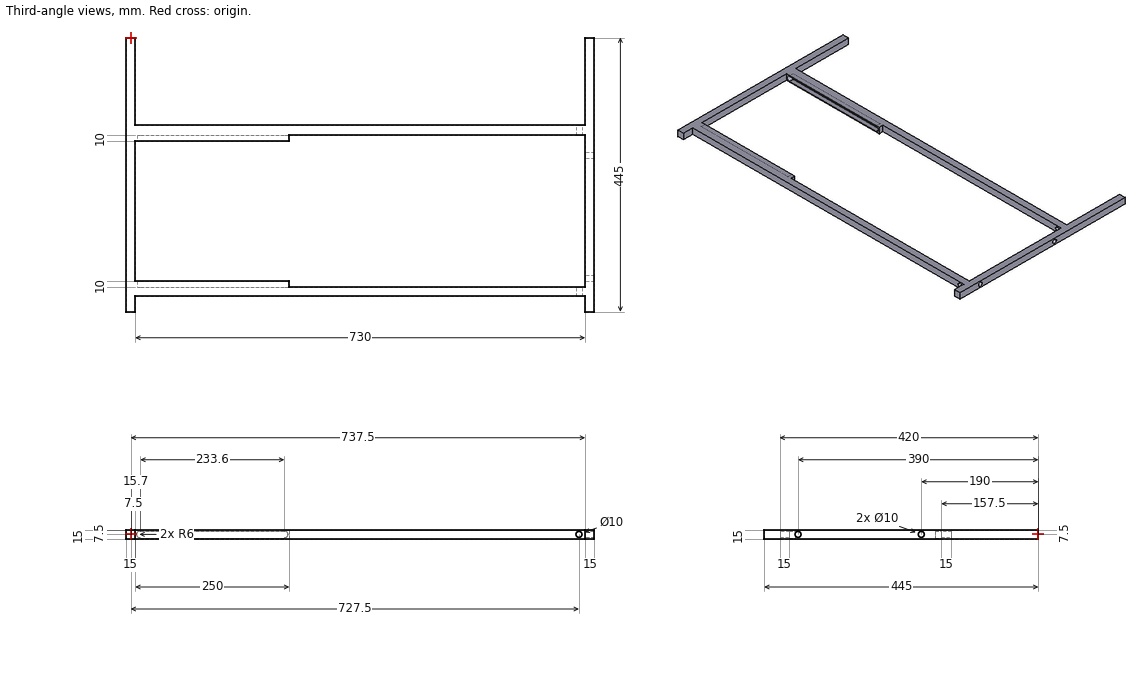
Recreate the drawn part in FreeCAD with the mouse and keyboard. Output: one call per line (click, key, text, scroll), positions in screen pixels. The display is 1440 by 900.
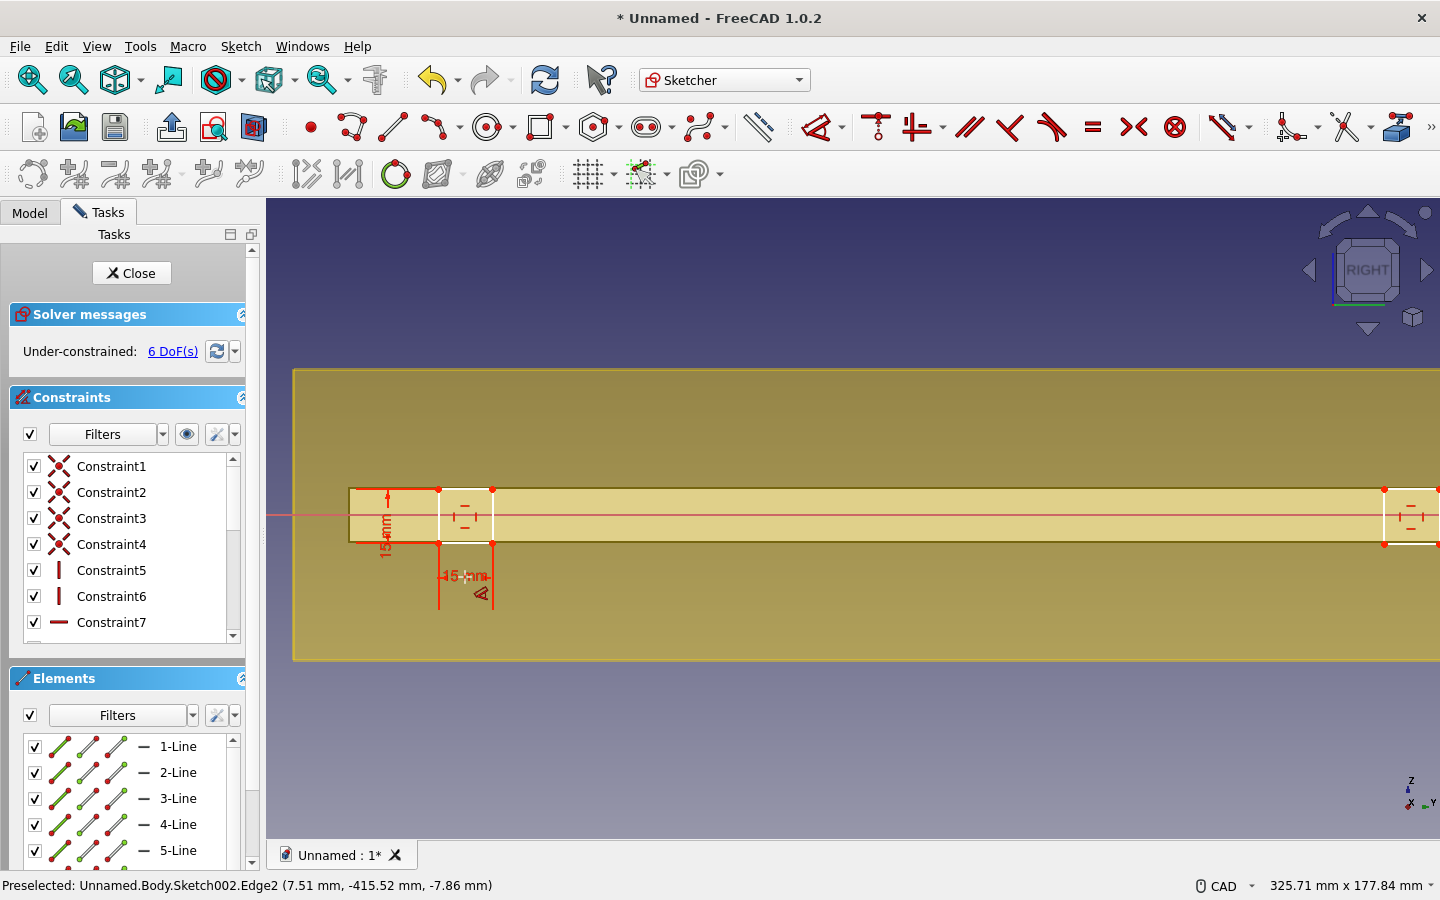
scroll(449, 521, down, 4)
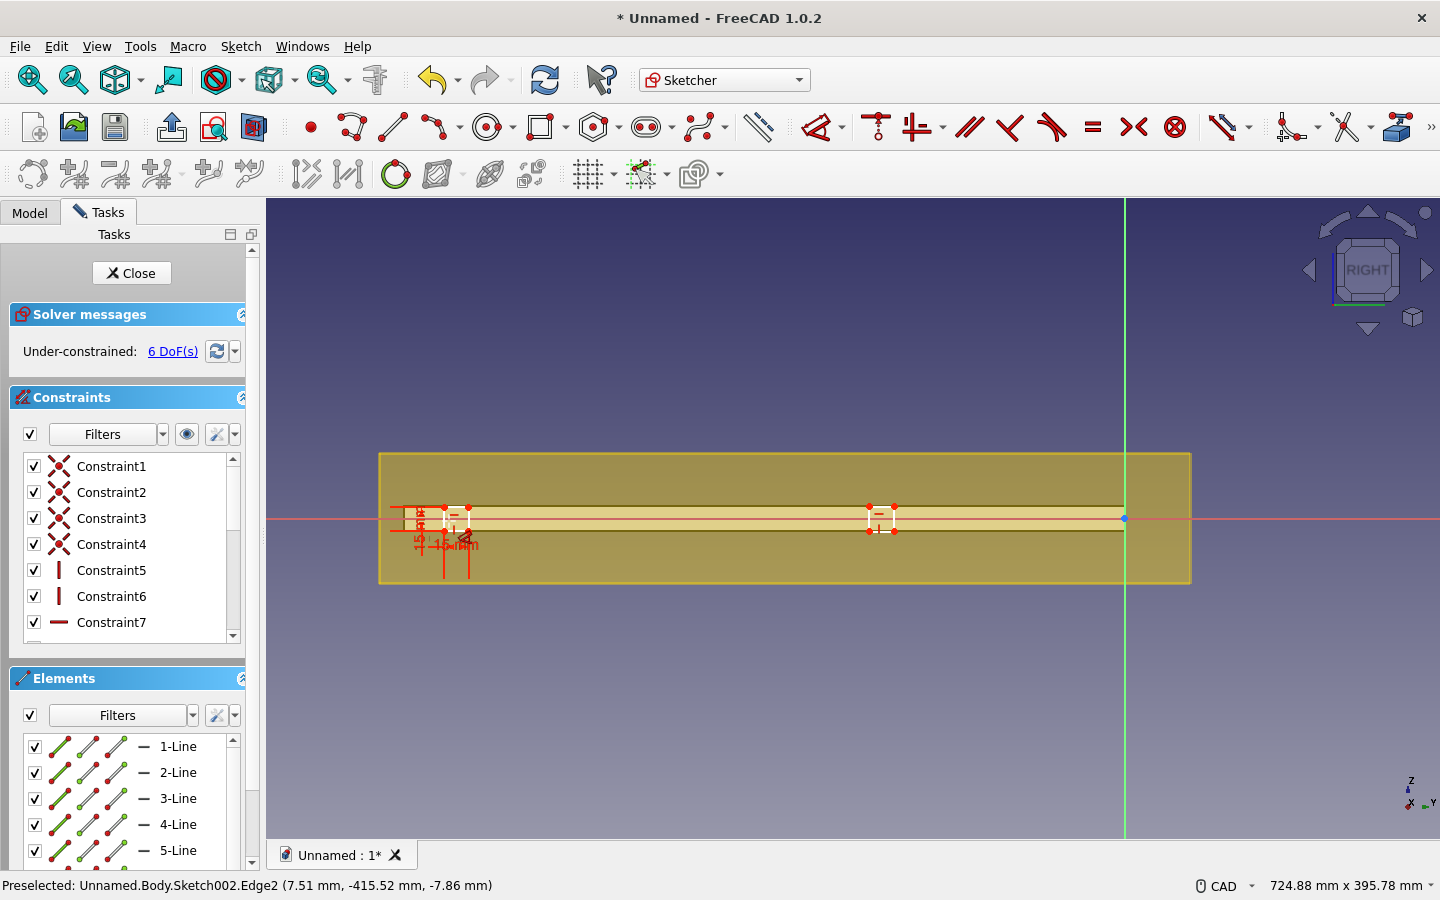
scroll(869, 514, up, 6)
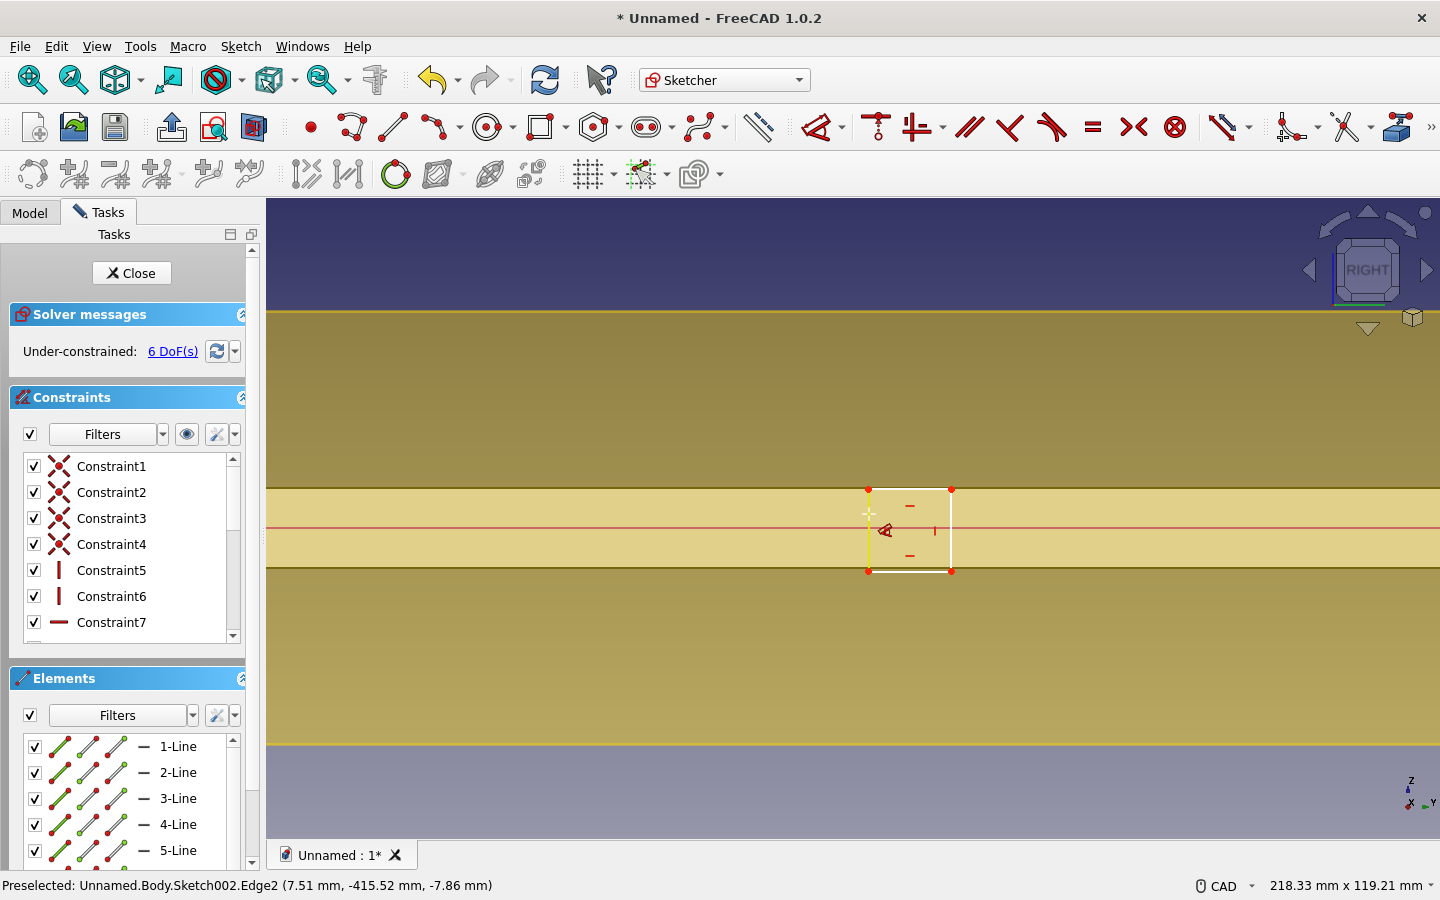
click(869, 514)
click(903, 512)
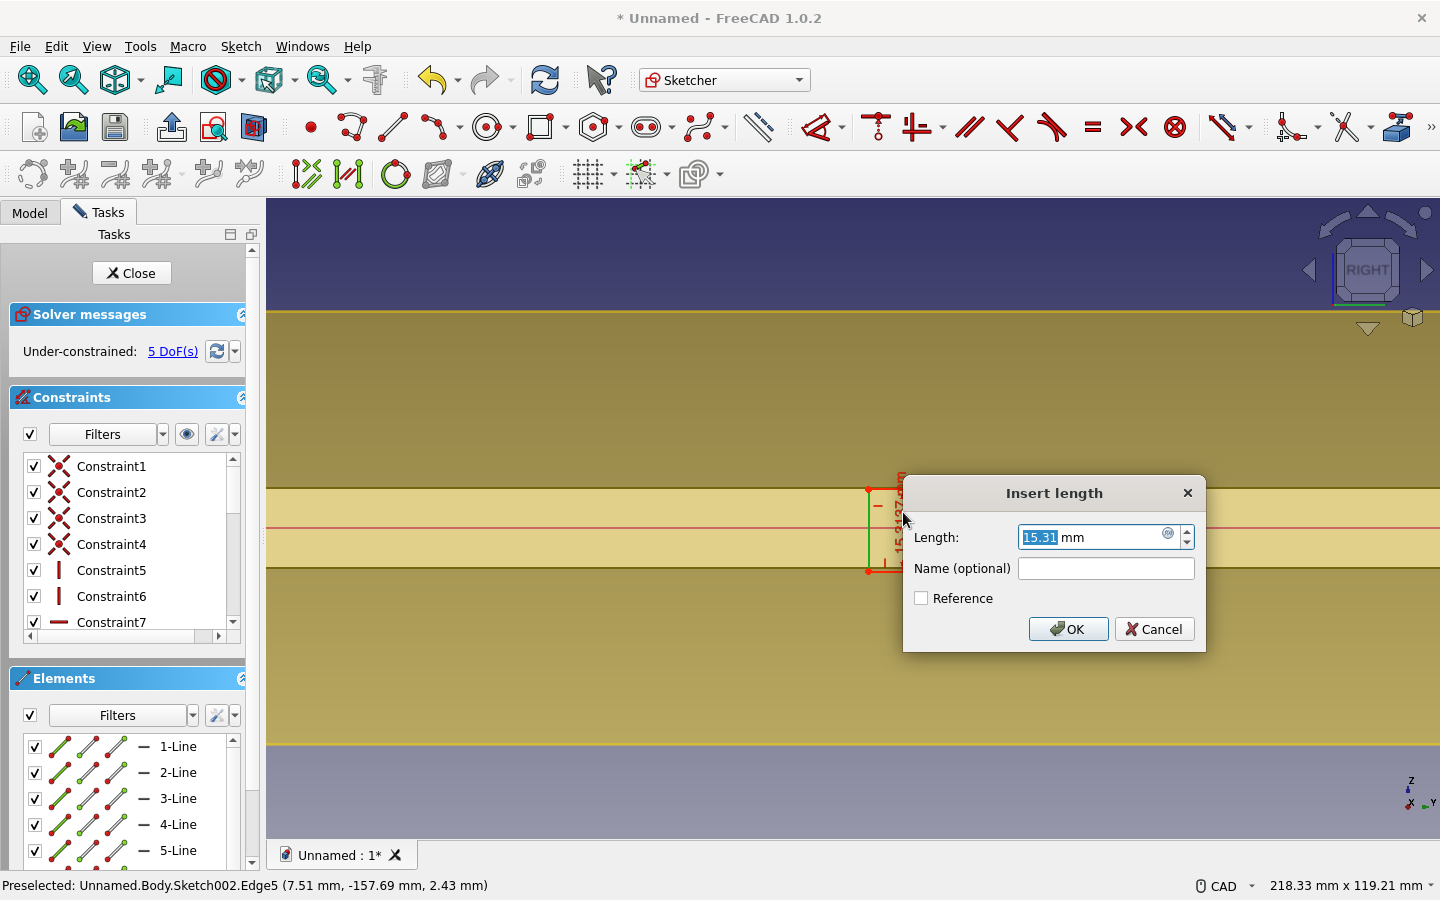
text(15)
key(Return)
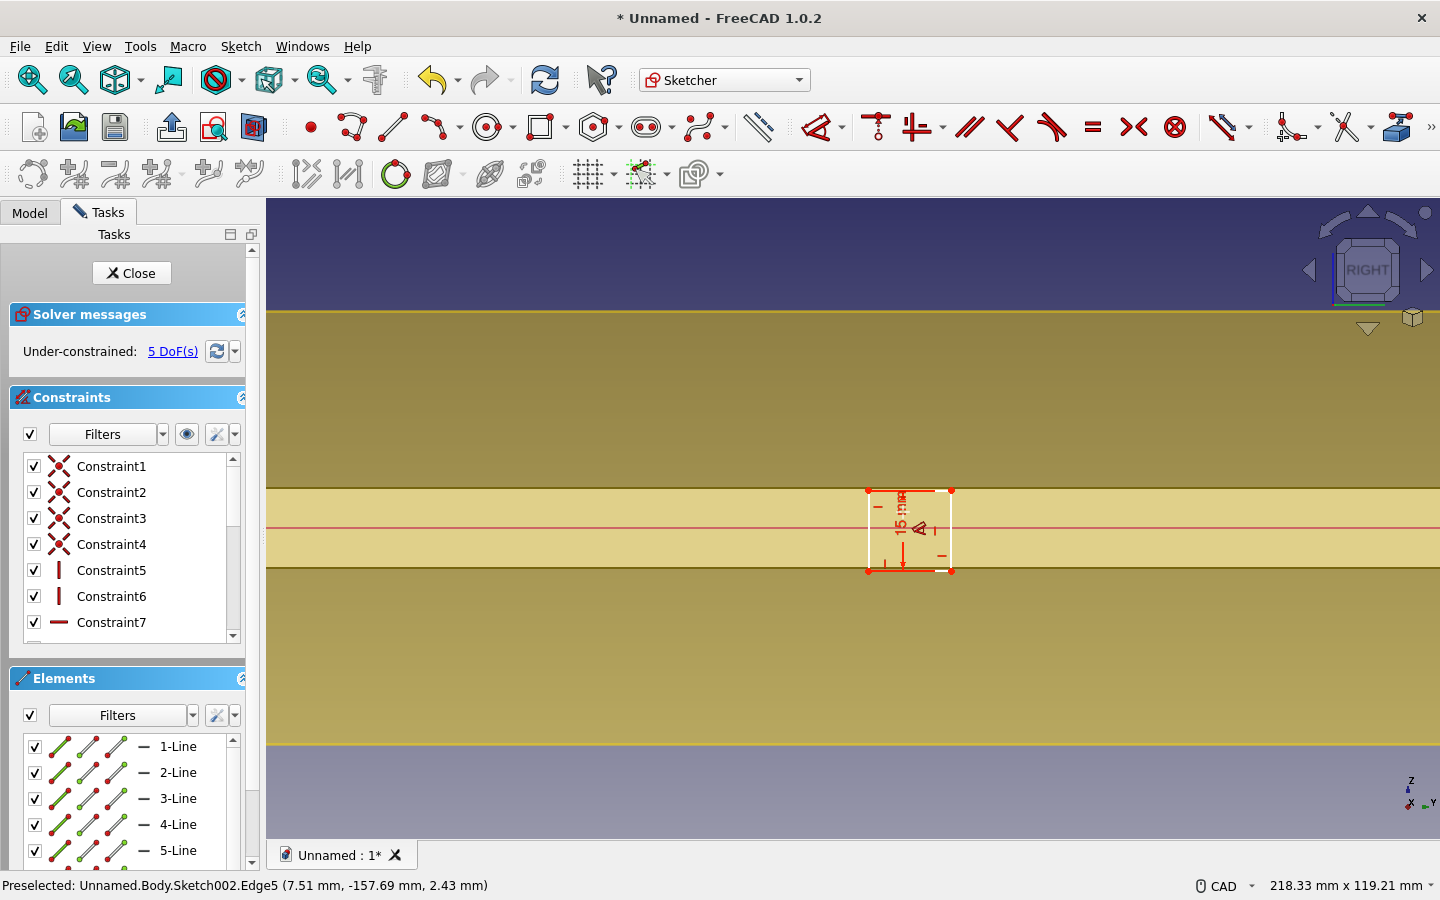
click(894, 571)
click(910, 605)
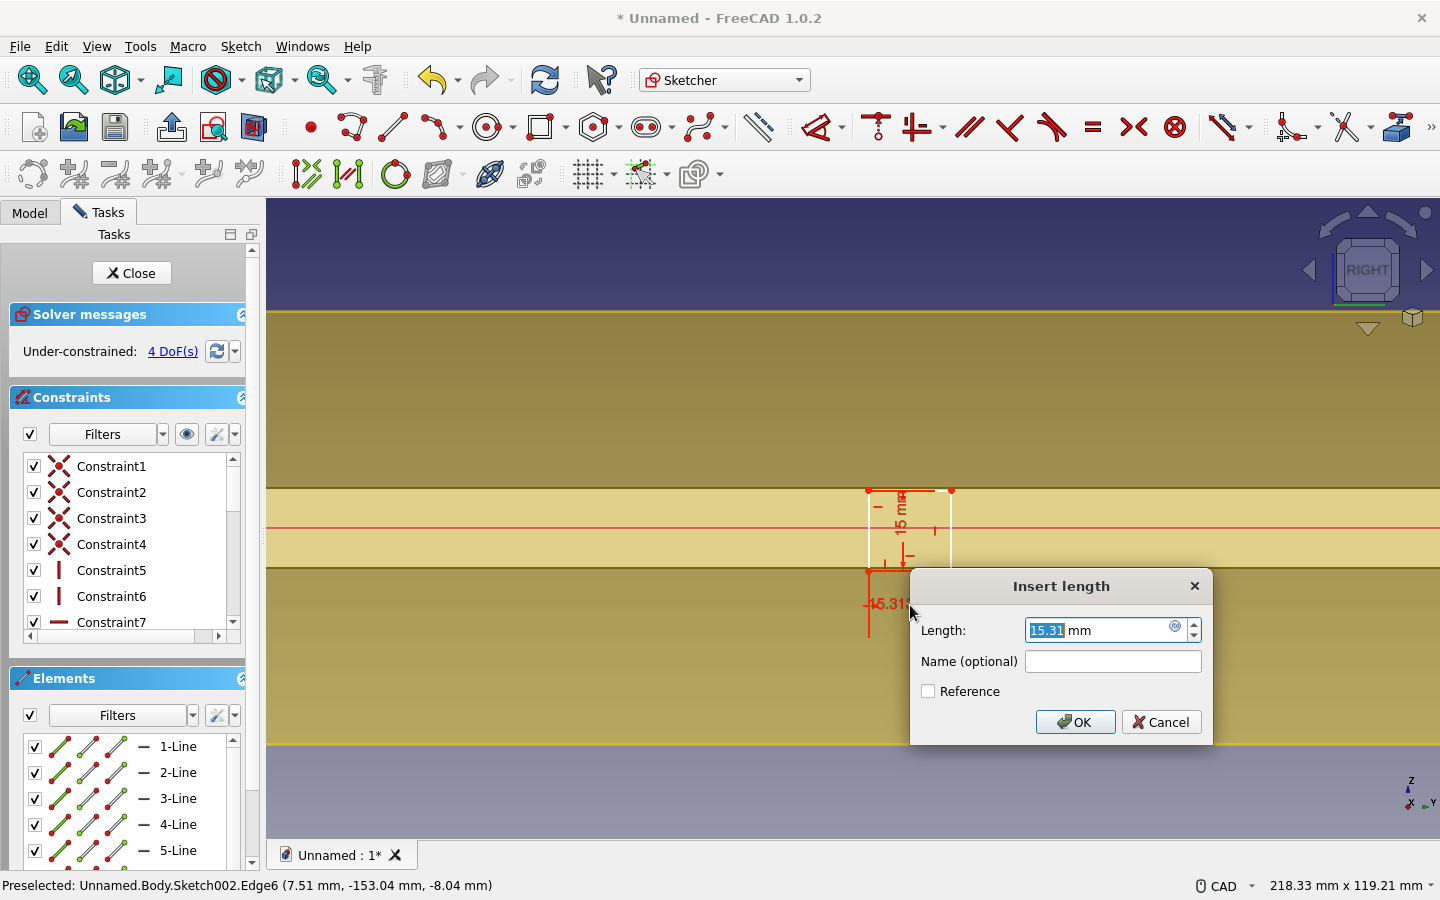
text(15)
key(Return)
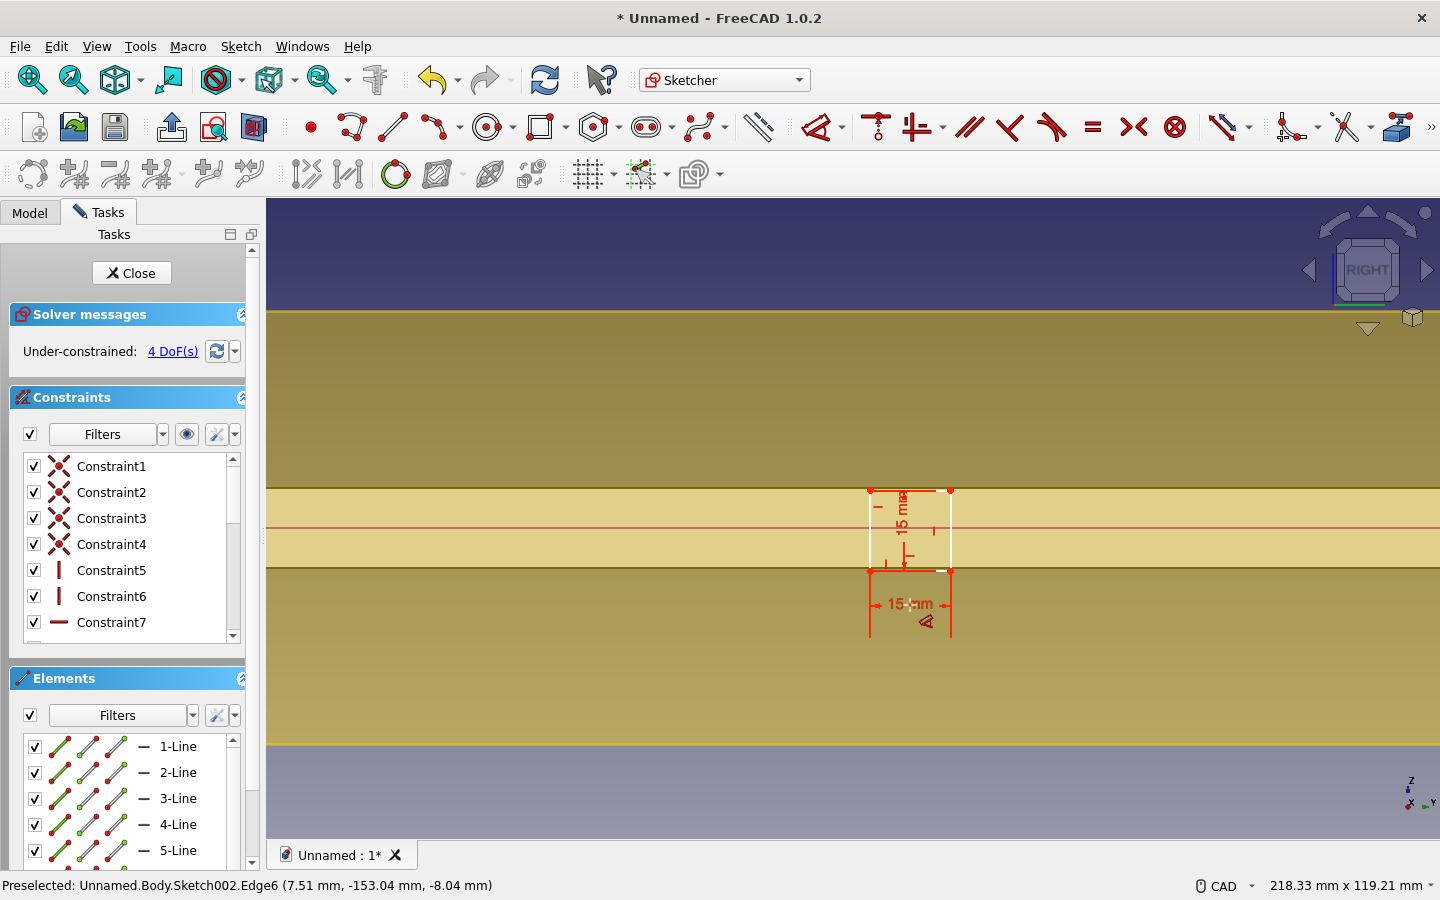
scroll(869, 514, down, 6)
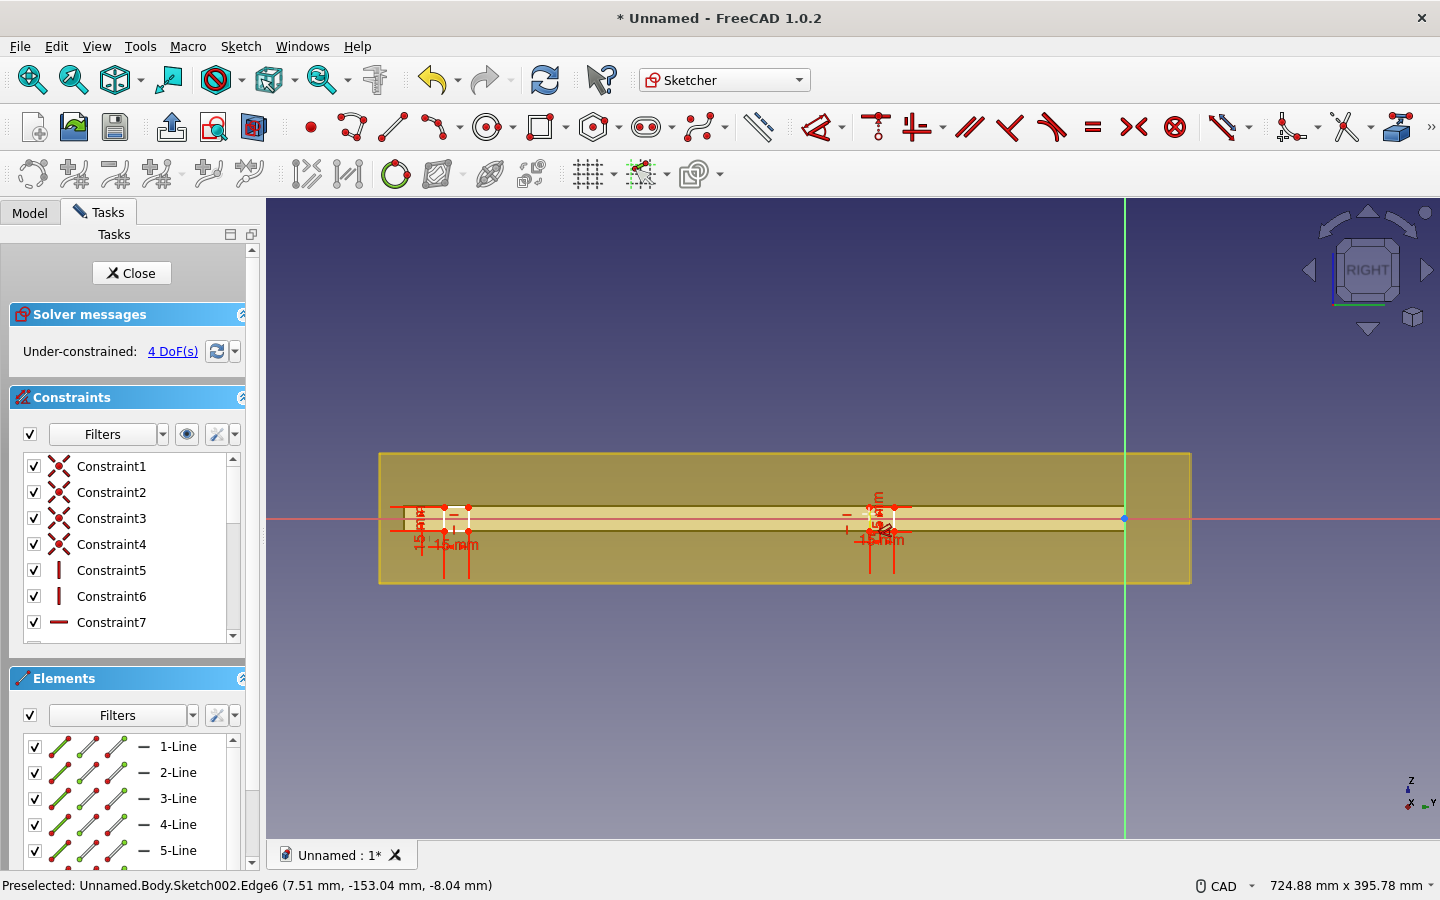
click(444, 507)
click(785, 473)